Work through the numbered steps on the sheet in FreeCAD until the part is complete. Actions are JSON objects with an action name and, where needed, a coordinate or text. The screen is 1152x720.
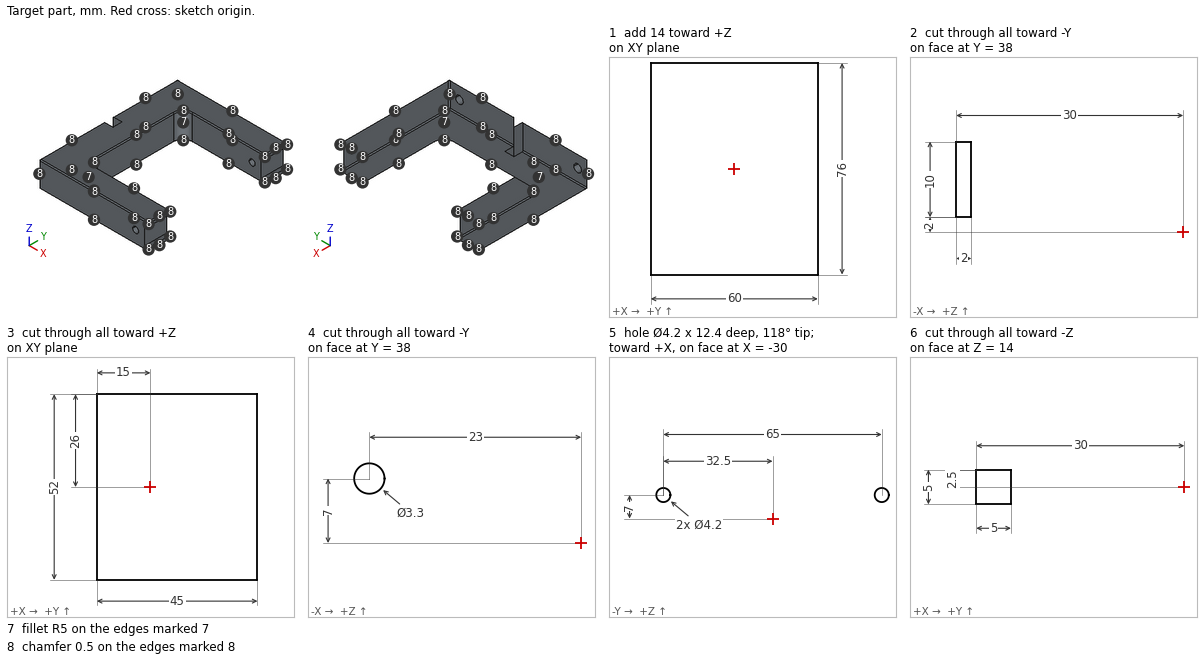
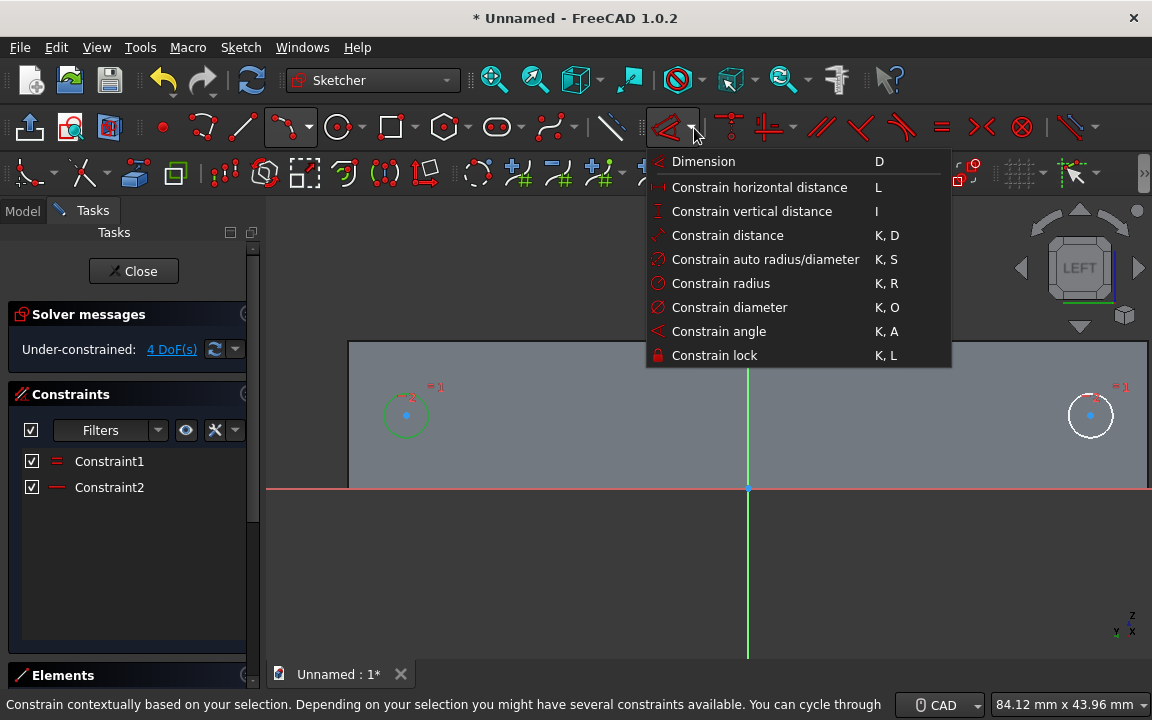
{"action": "left_click", "coordinate": [799, 307]}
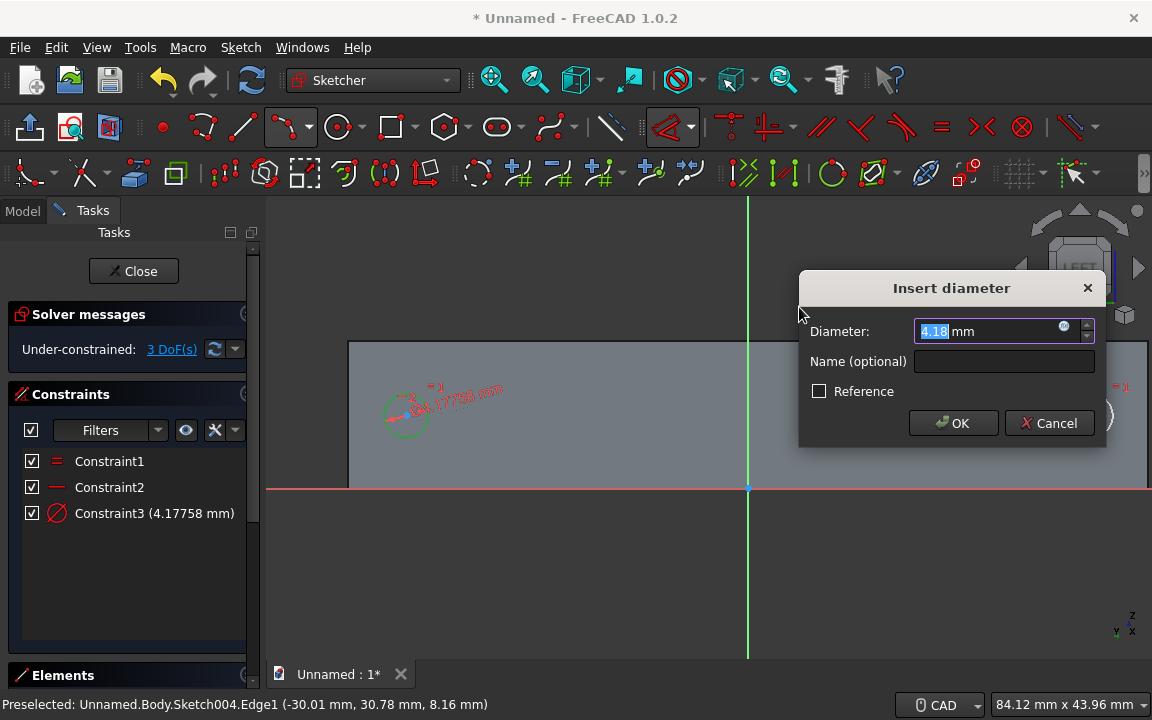
{"action": "type", "text": "4.2"}
{"action": "key", "text": "Return"}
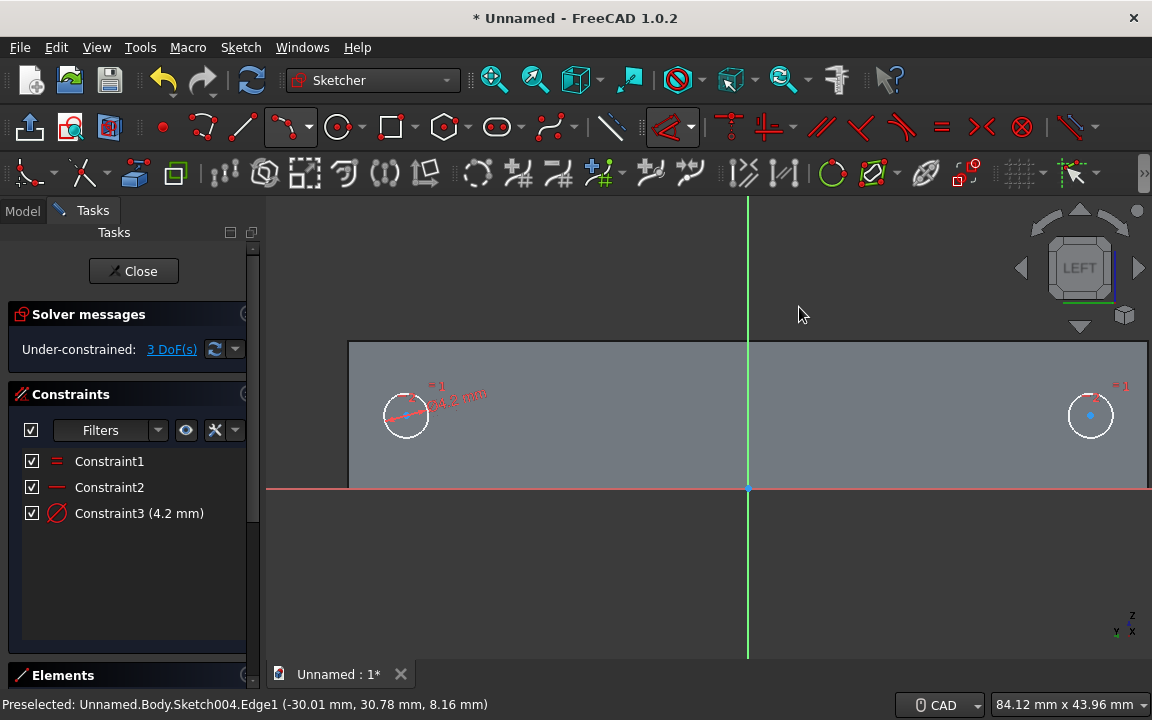
{"action": "left_click", "coordinate": [406, 416]}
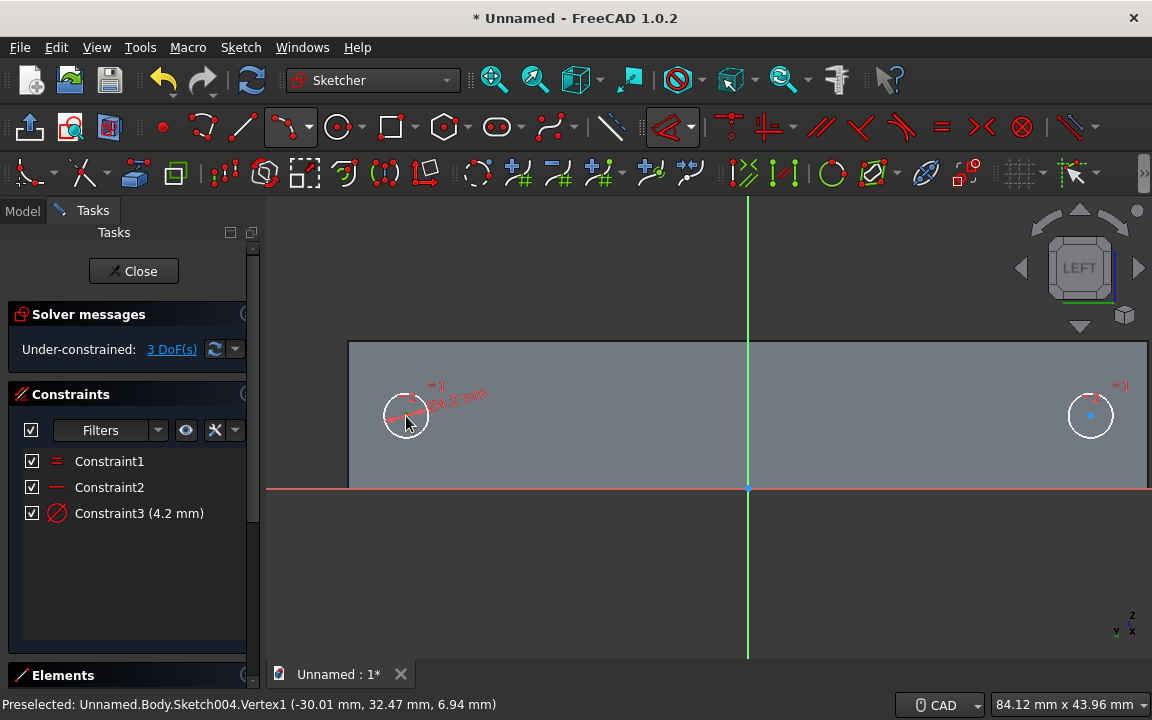
{"action": "key", "text": "i"}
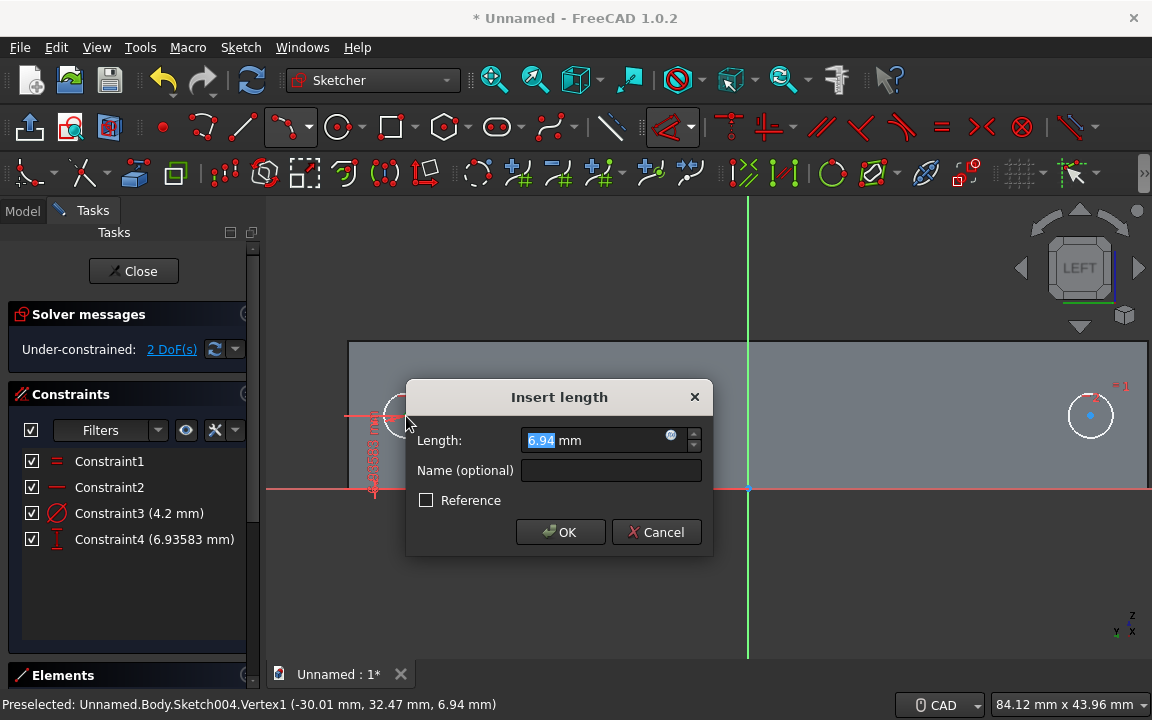
{"action": "type", "text": "7"}
{"action": "key", "text": "Return"}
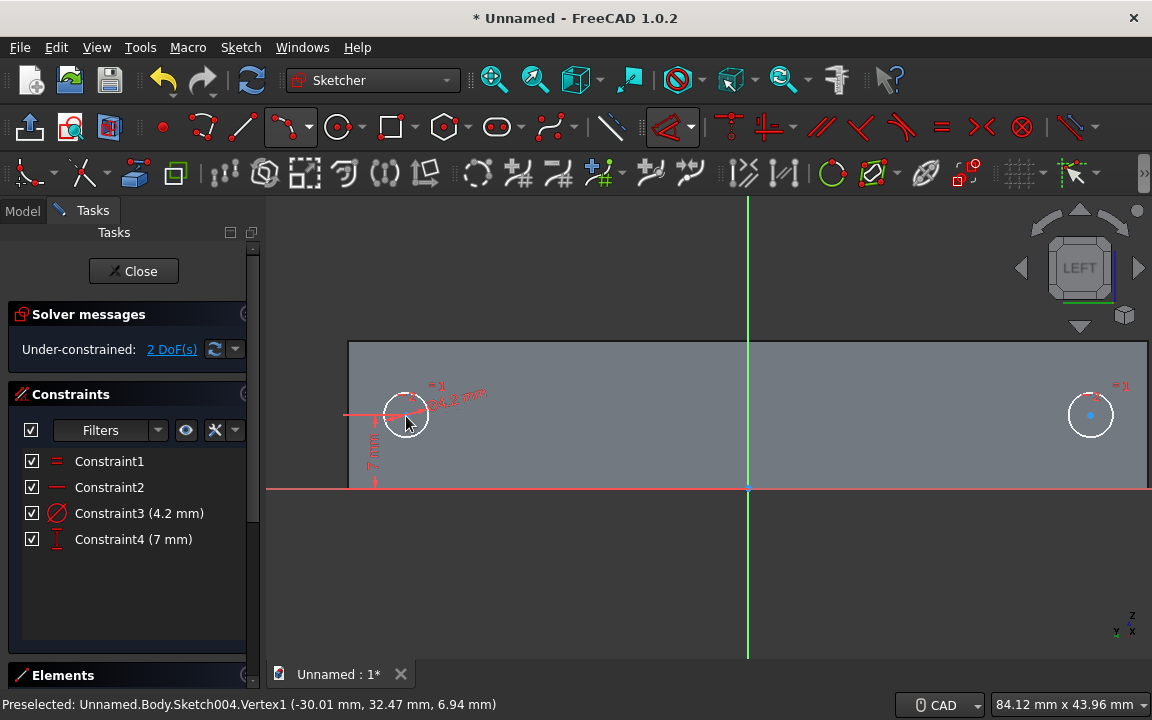
{"action": "left_click", "coordinate": [406, 415]}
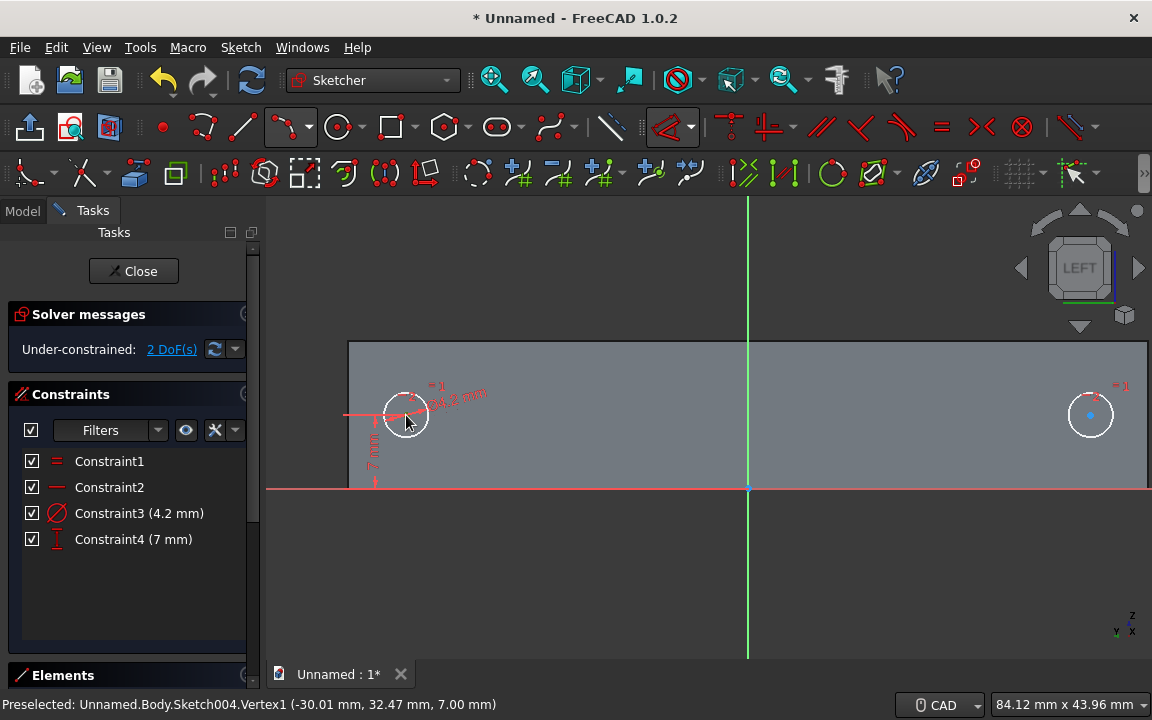
{"action": "scroll", "coordinate": [421, 400], "scroll_direction": "down", "scroll_amount": 2}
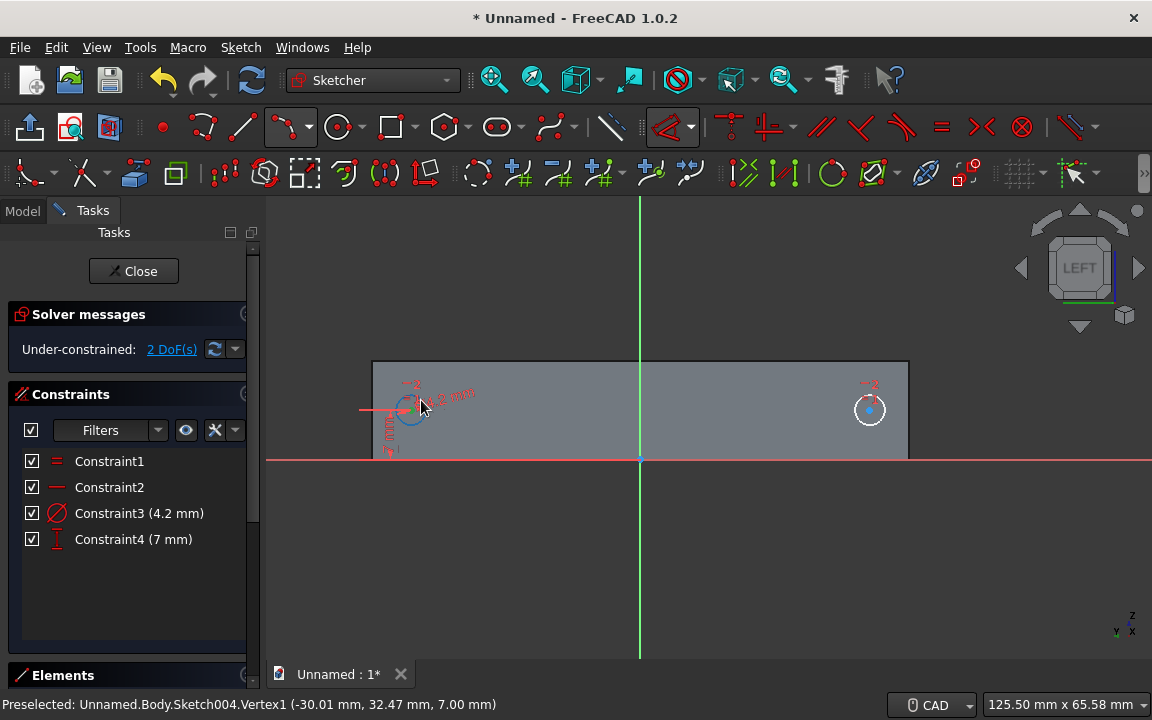
{"action": "left_click", "coordinate": [870, 410]}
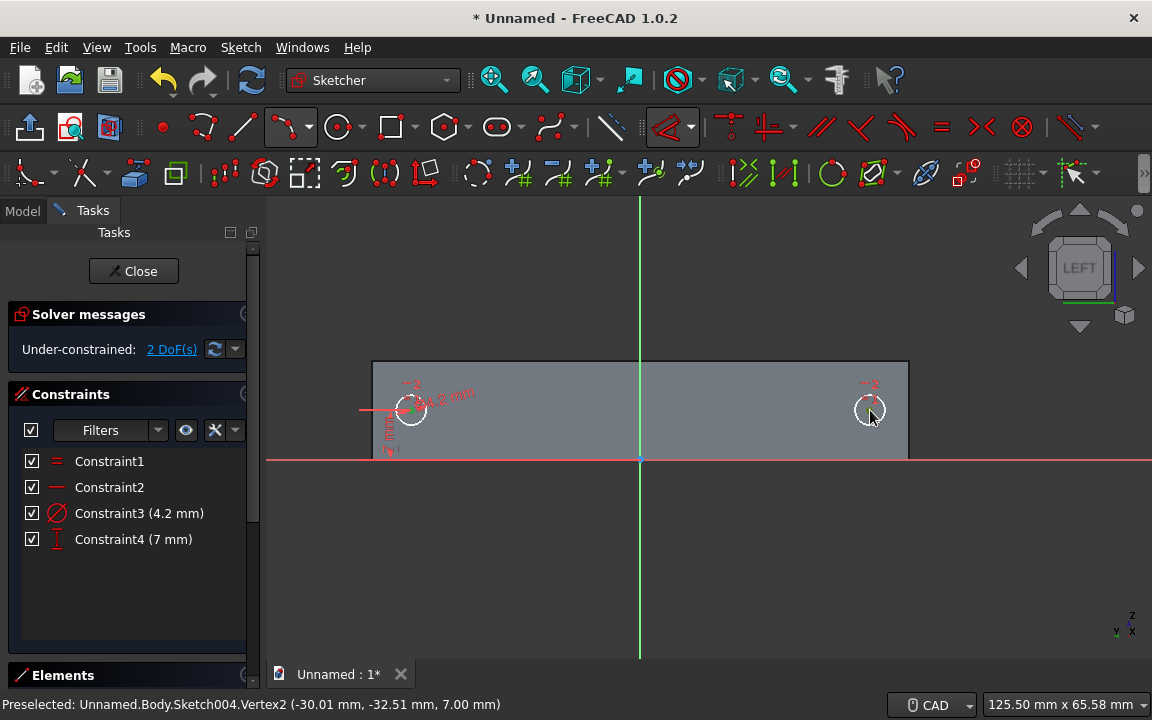
{"action": "key", "text": "l"}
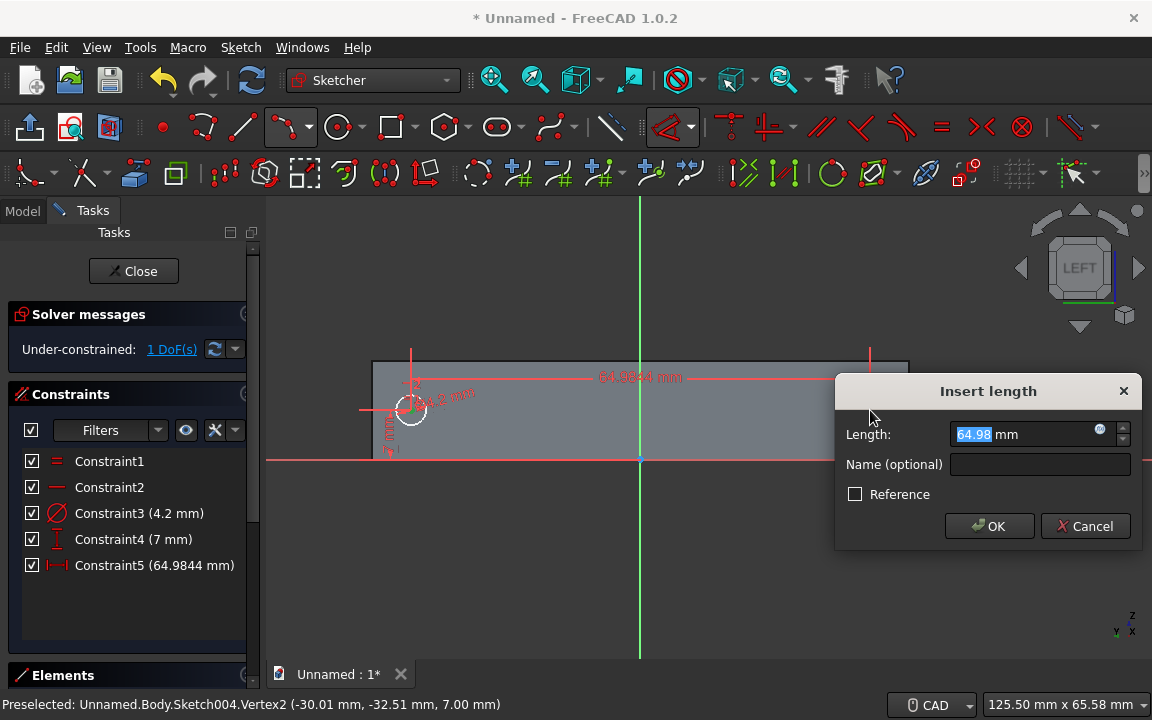
{"action": "type", "text": "65"}
{"action": "key", "text": "Return"}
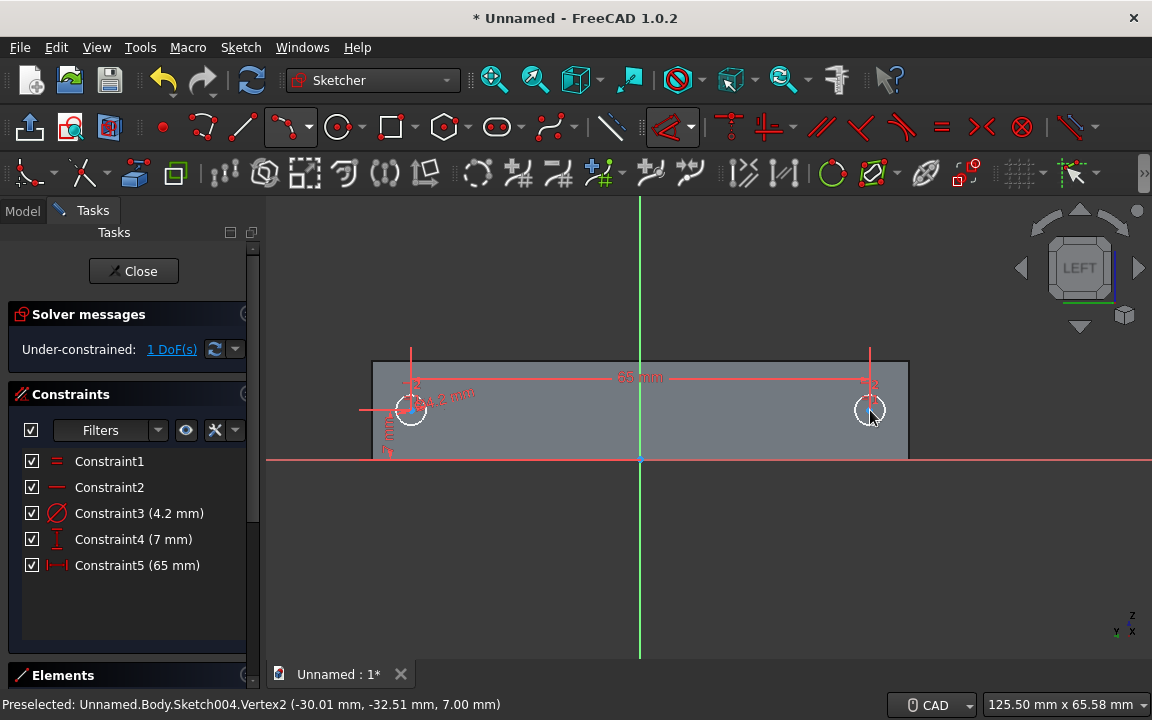
{"action": "left_click", "coordinate": [411, 410]}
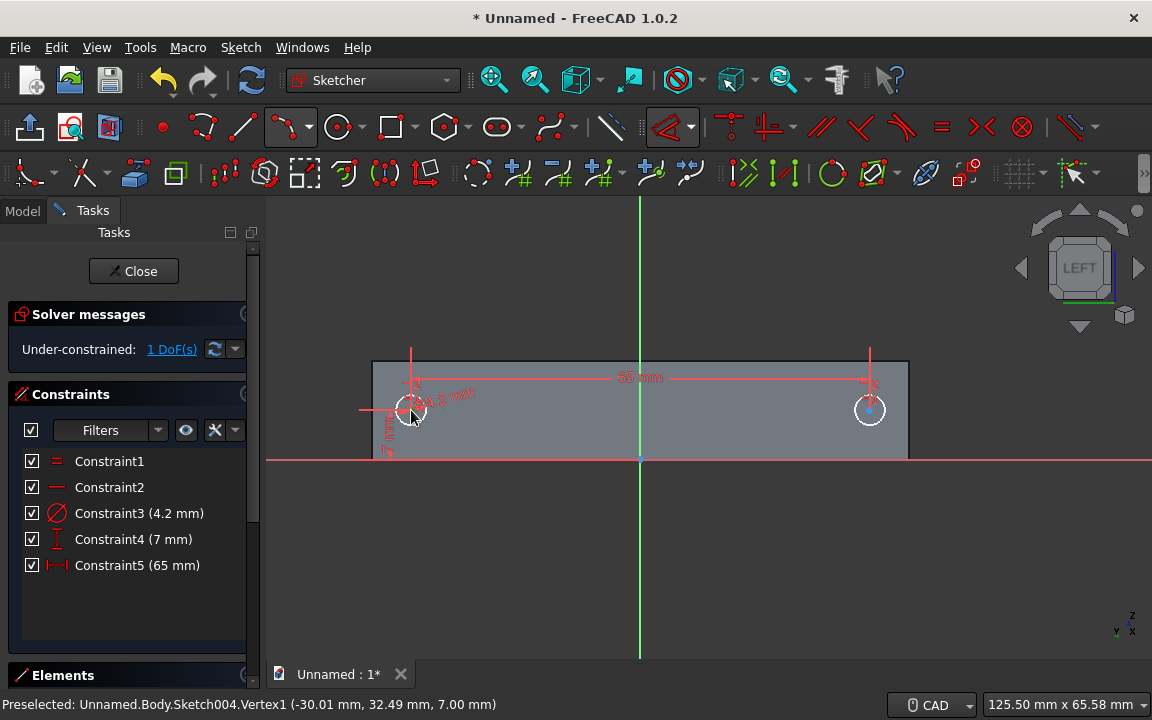
{"action": "key", "text": "l"}